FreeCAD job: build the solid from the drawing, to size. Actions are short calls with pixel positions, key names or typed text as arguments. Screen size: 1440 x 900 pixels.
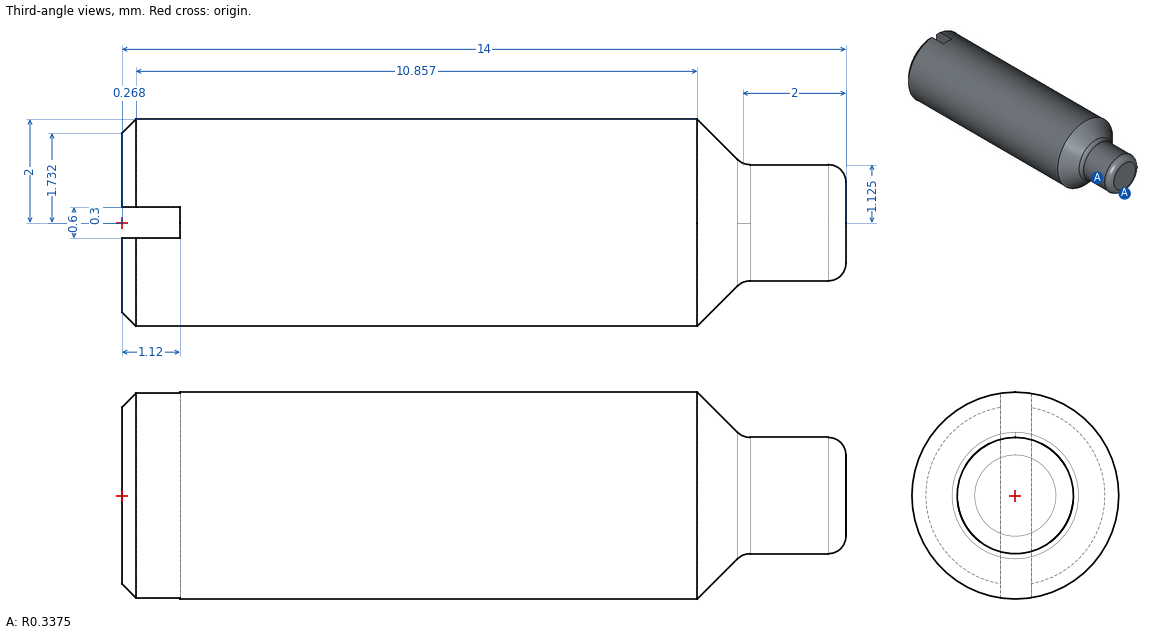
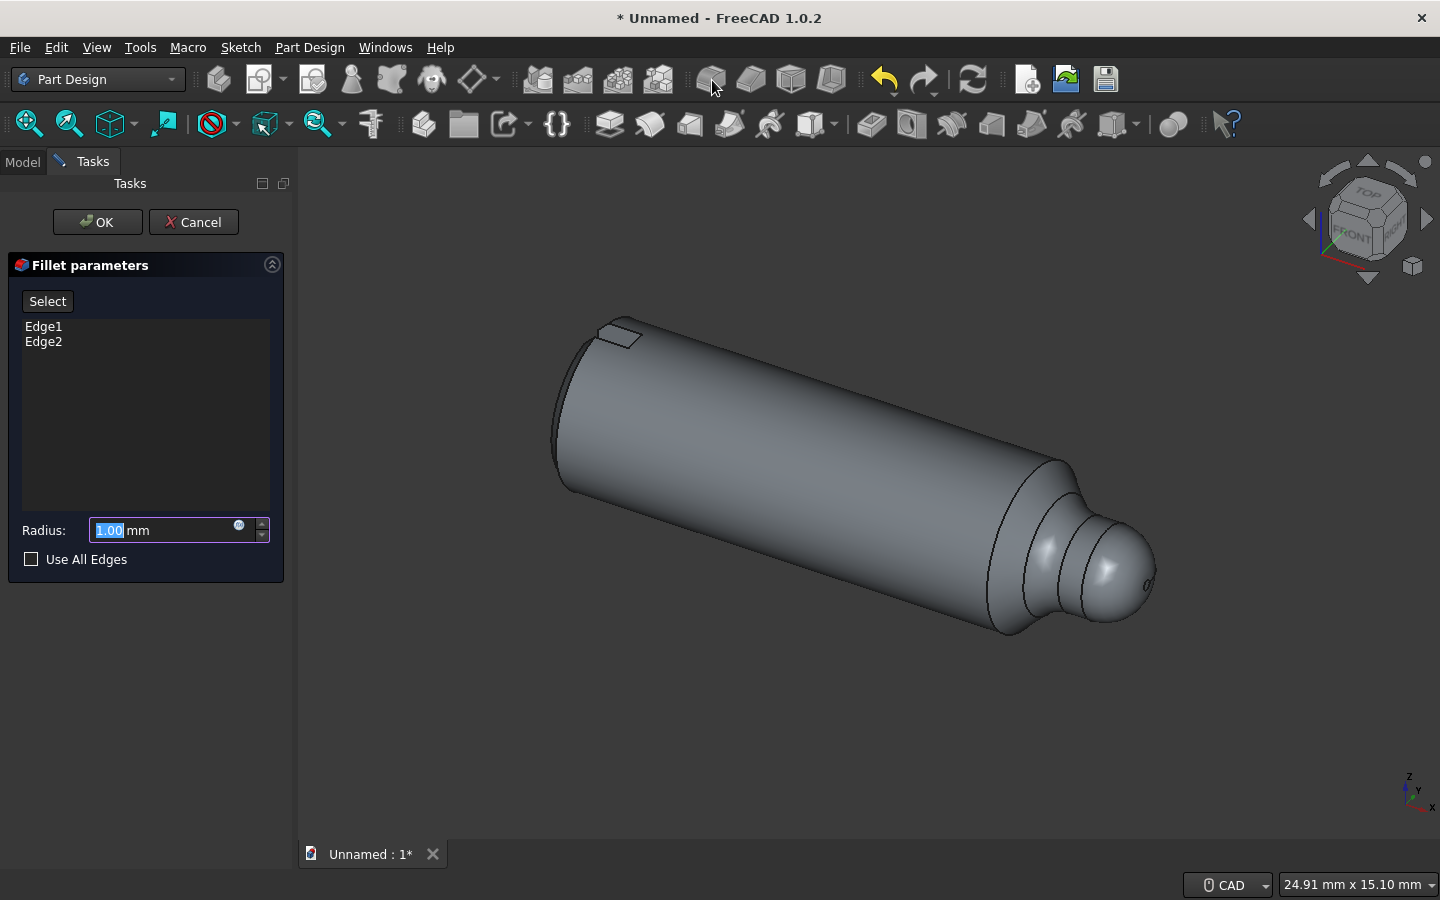
text(0.3375)
key(Tab)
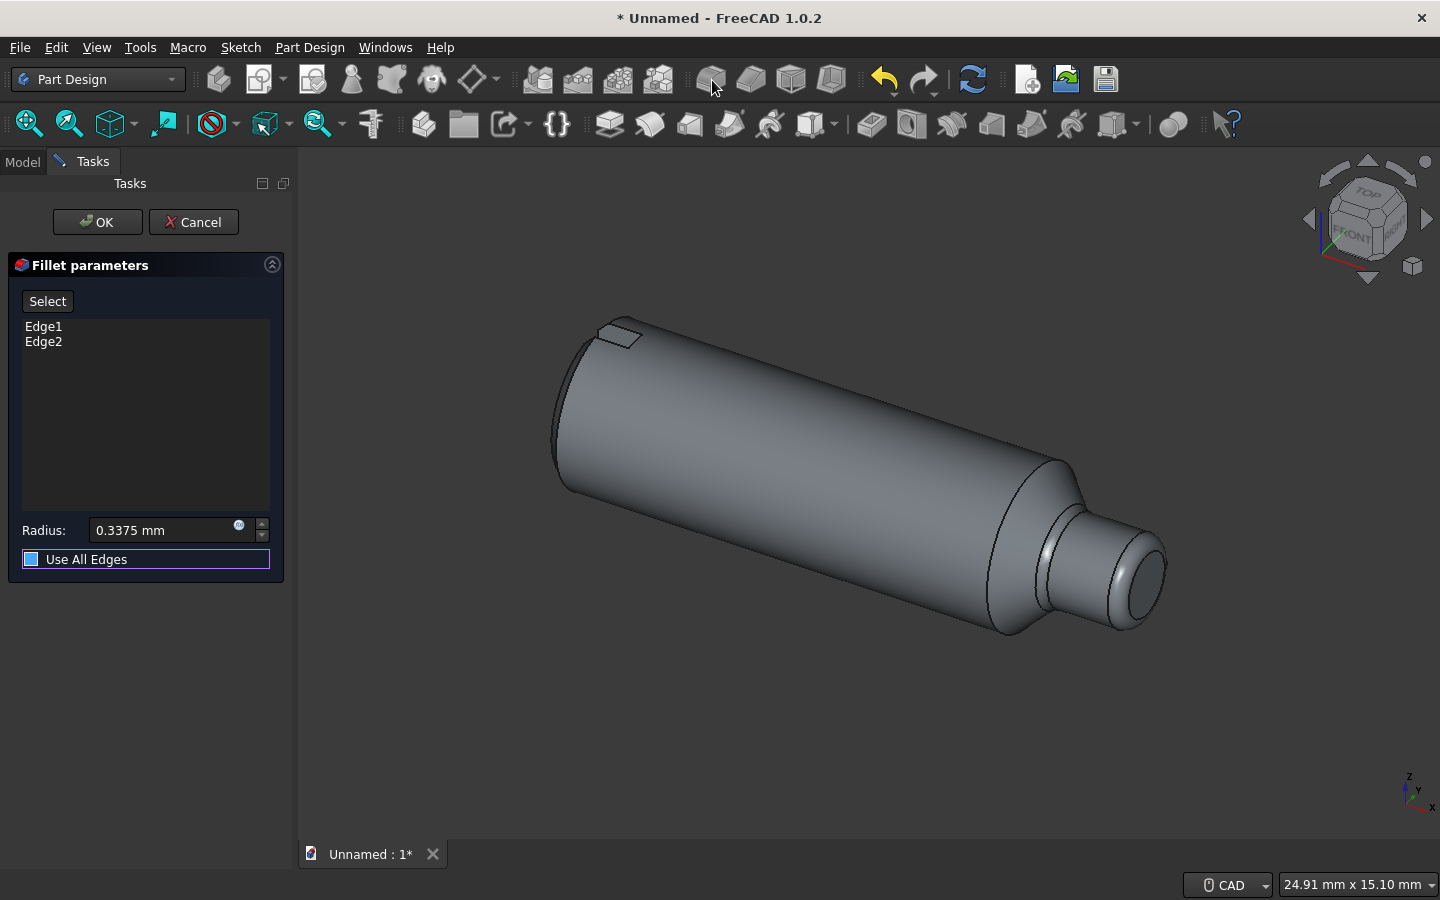
click(98, 222)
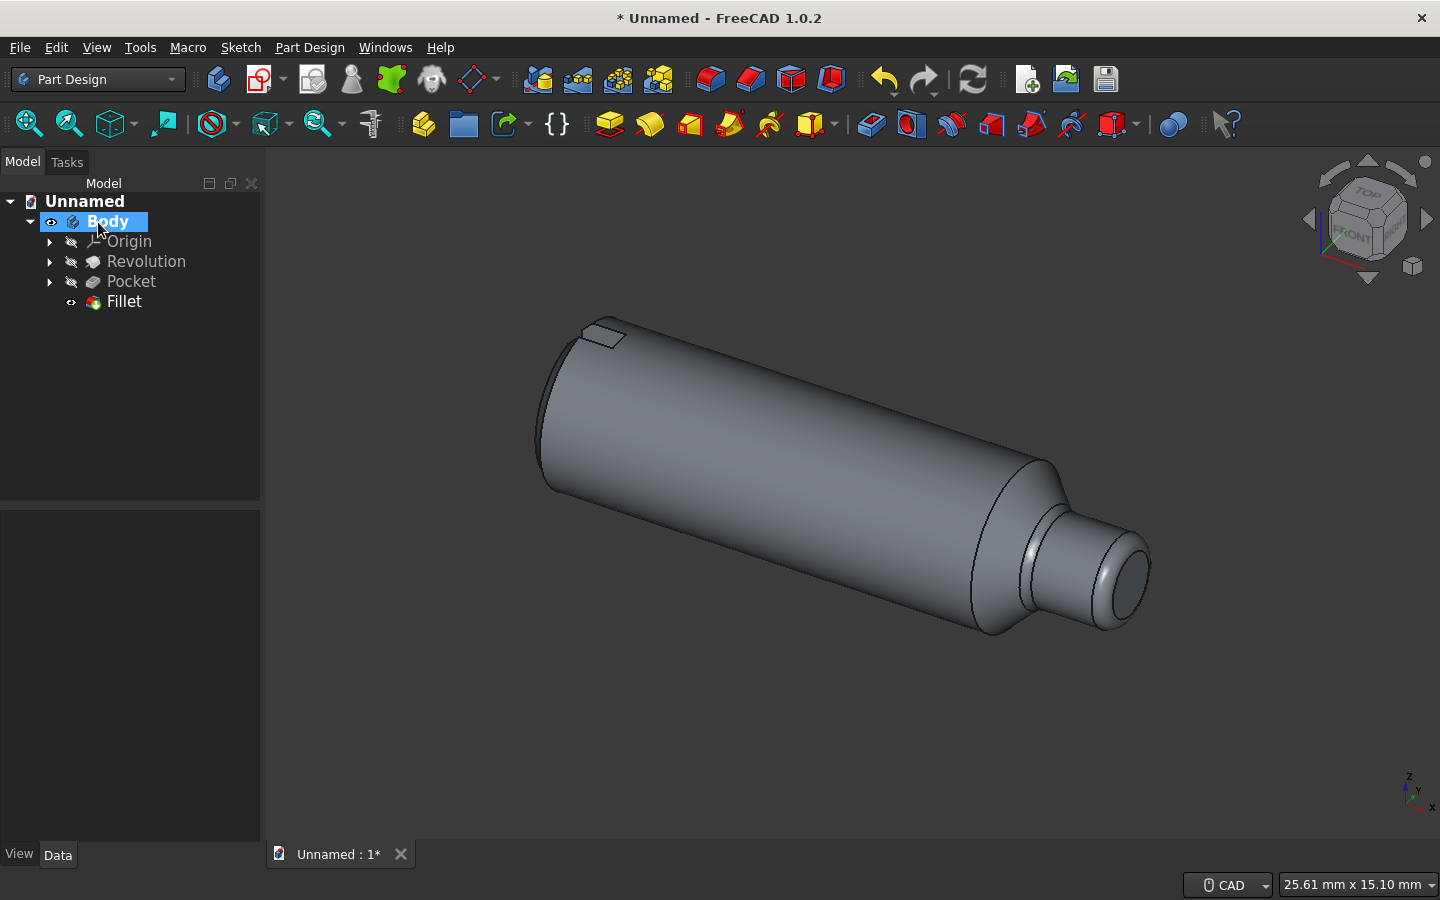
key(0)